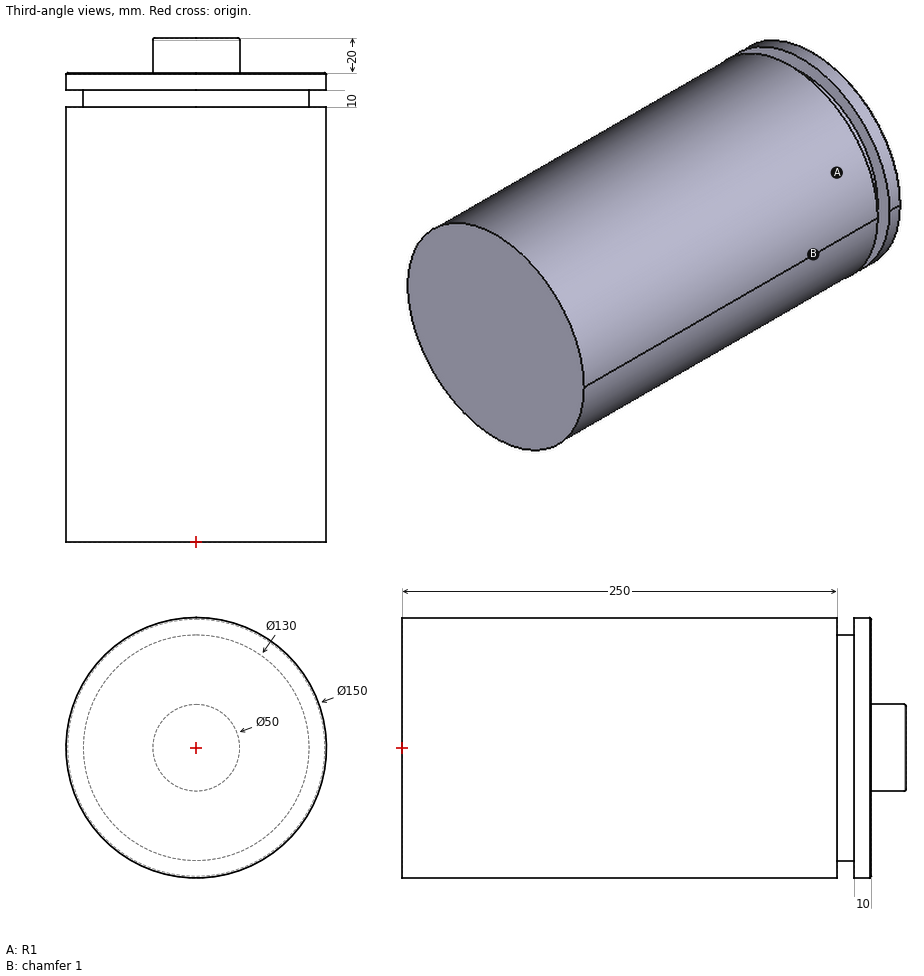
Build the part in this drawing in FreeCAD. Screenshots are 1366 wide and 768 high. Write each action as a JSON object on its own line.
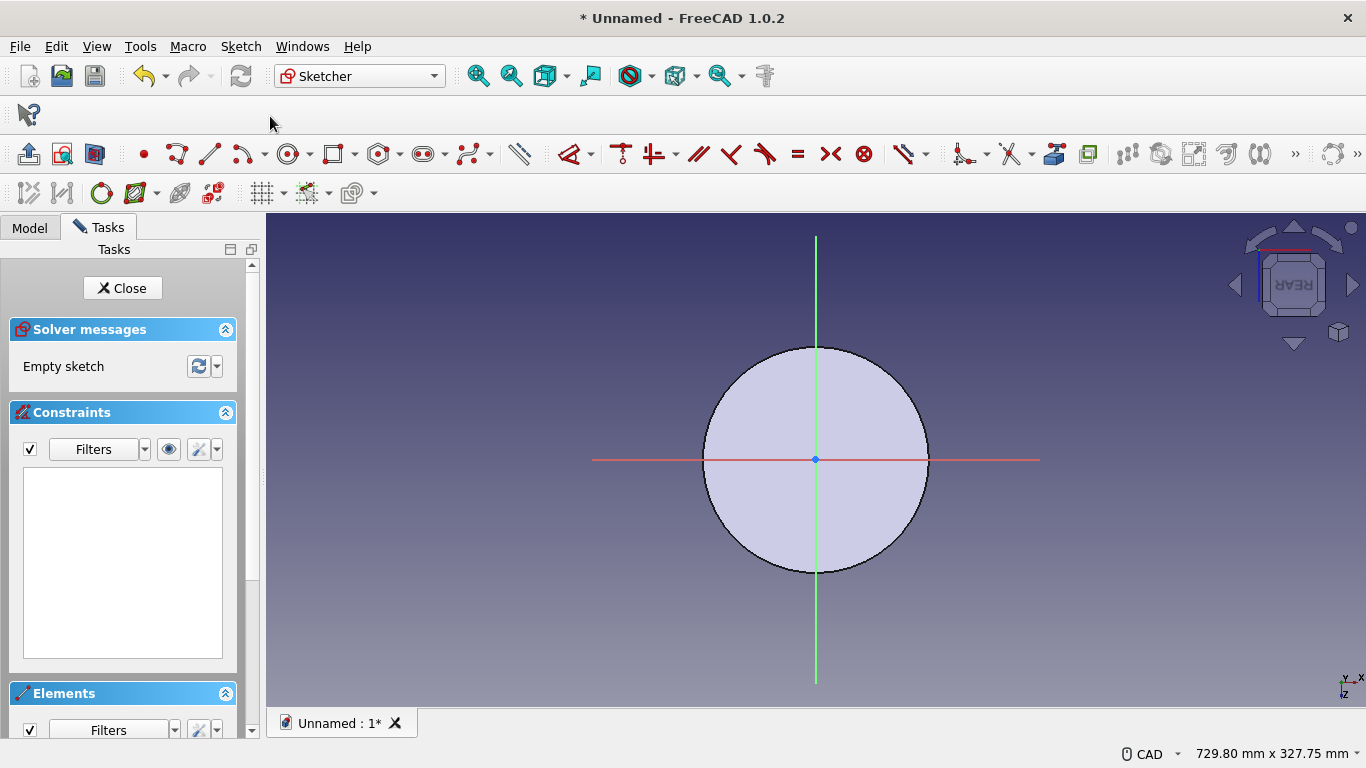
{"action": "scroll", "coordinate": [838, 460], "scroll_direction": "up", "scroll_amount": 7}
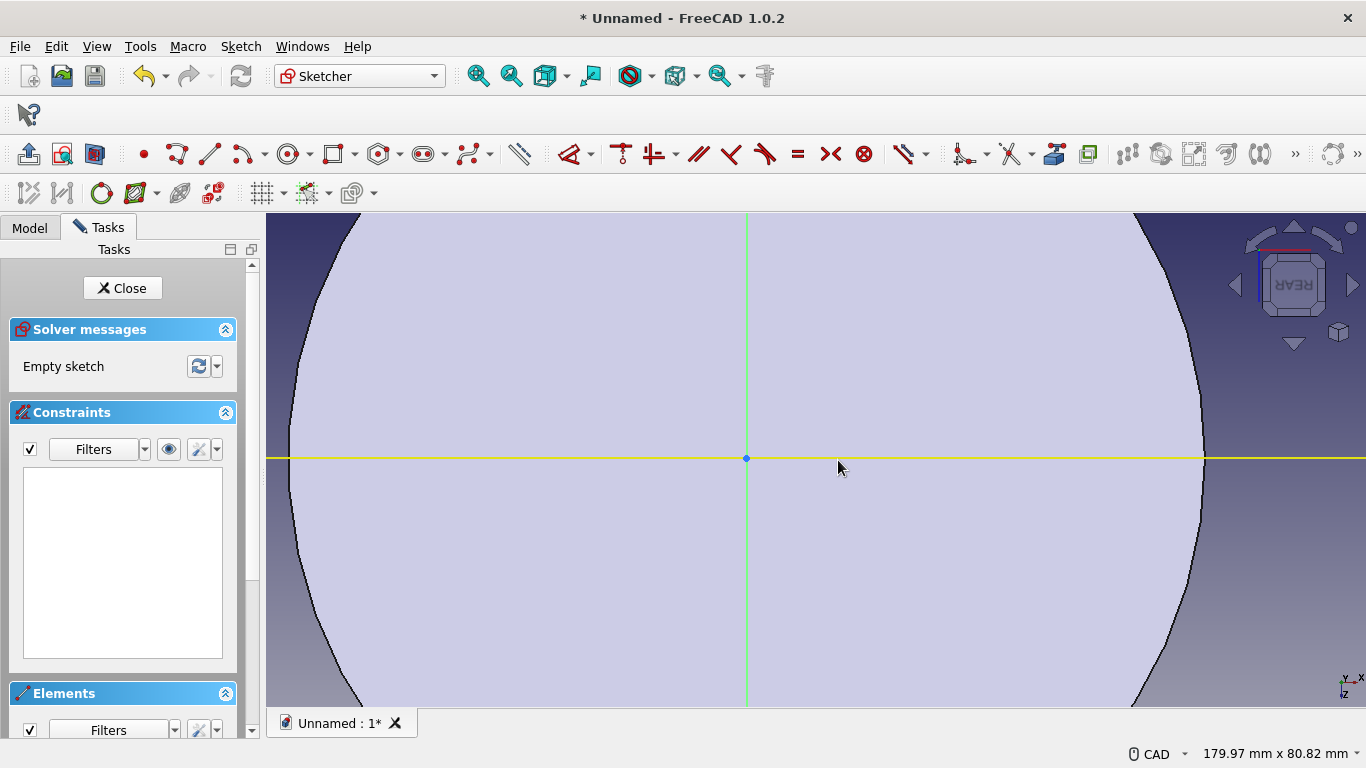
{"action": "key", "text": "g c"}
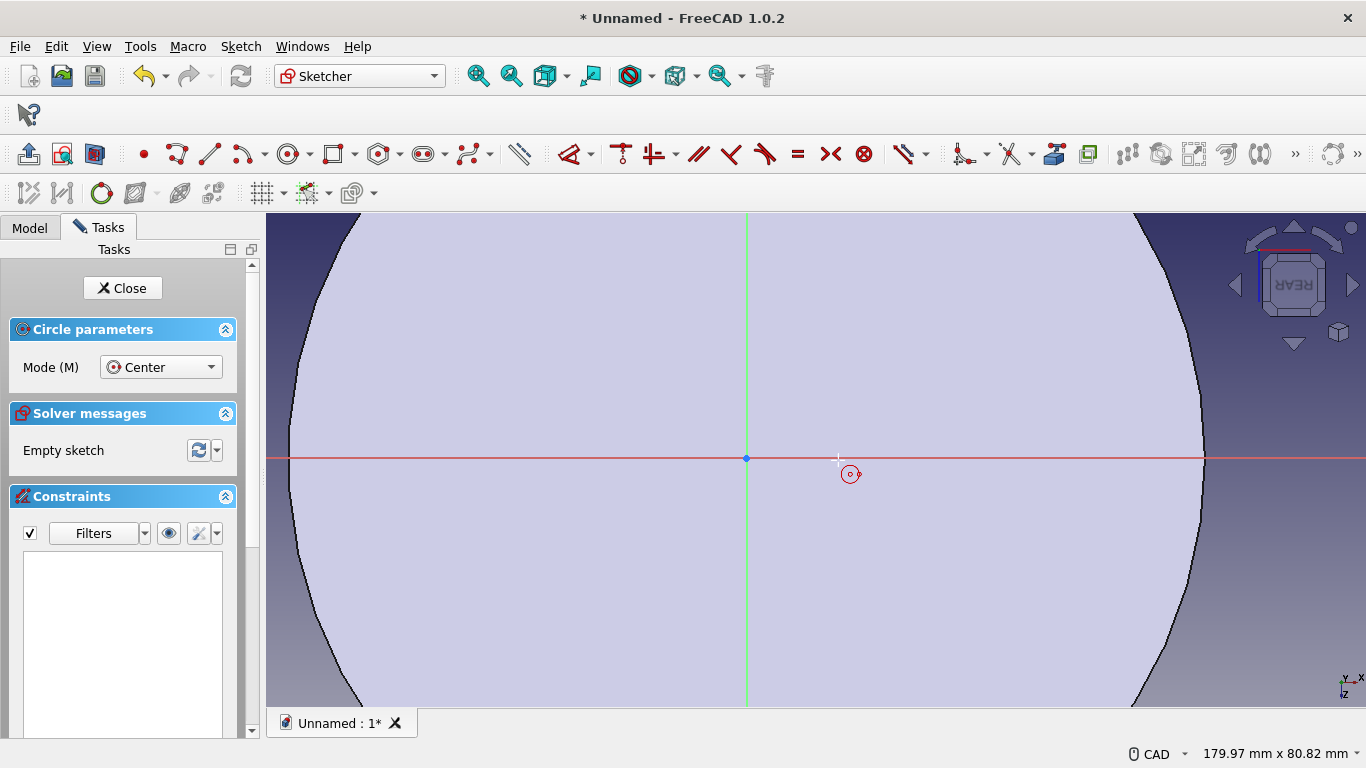
{"action": "left_click", "coordinate": [747, 458]}
{"action": "mouse_move", "coordinate": [855, 350]}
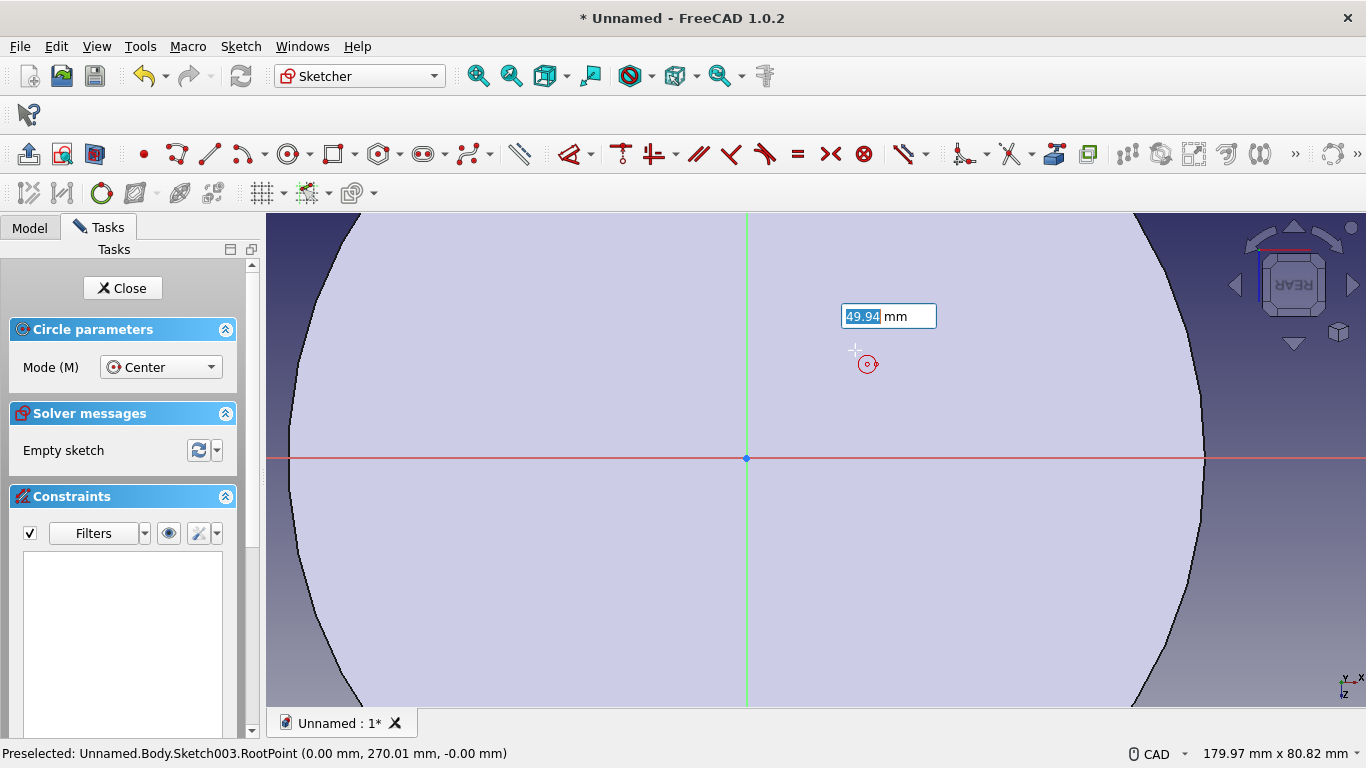
{"action": "type", "text": "50"}
{"action": "key", "text": "Return"}
{"action": "key", "text": "Escape"}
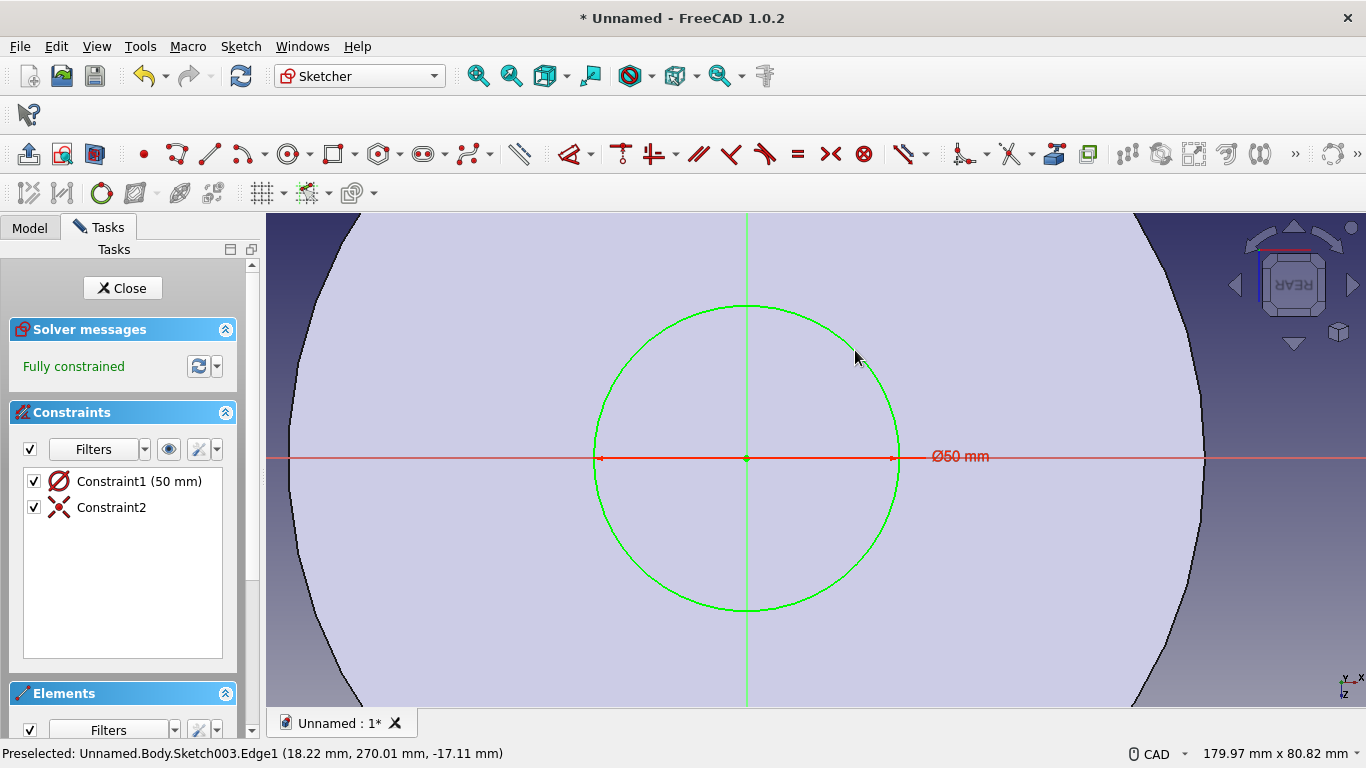
{"action": "left_click", "coordinate": [123, 288]}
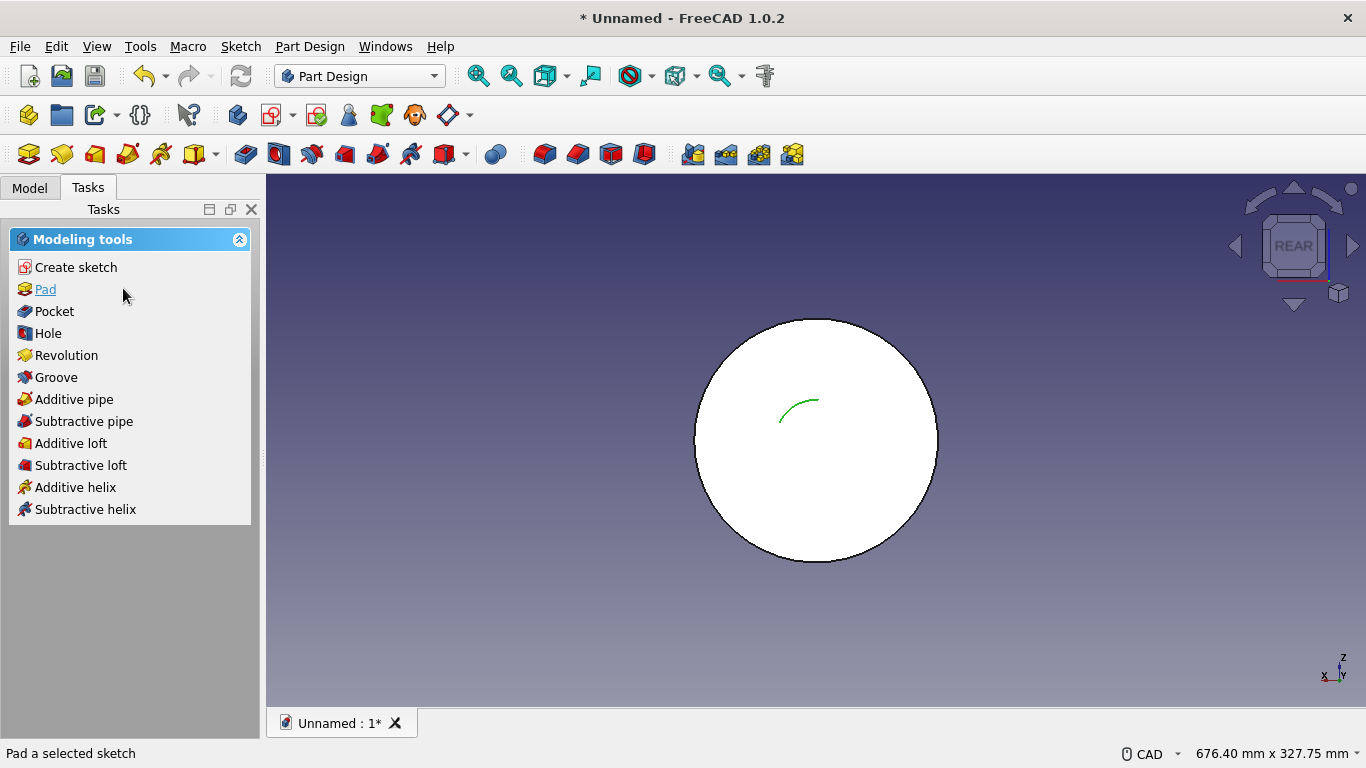
{"action": "left_click", "coordinate": [29, 154]}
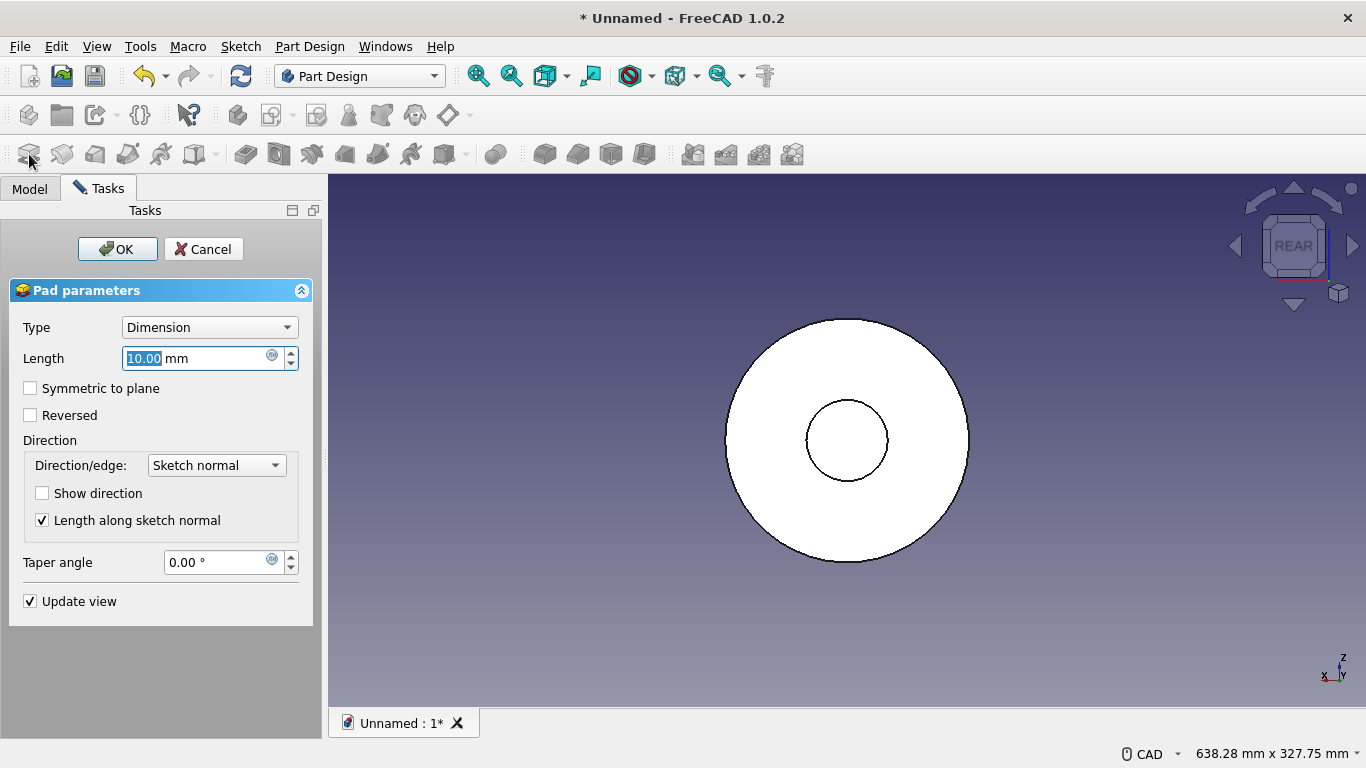
{"action": "type", "text": "20"}
{"action": "key", "text": "Tab"}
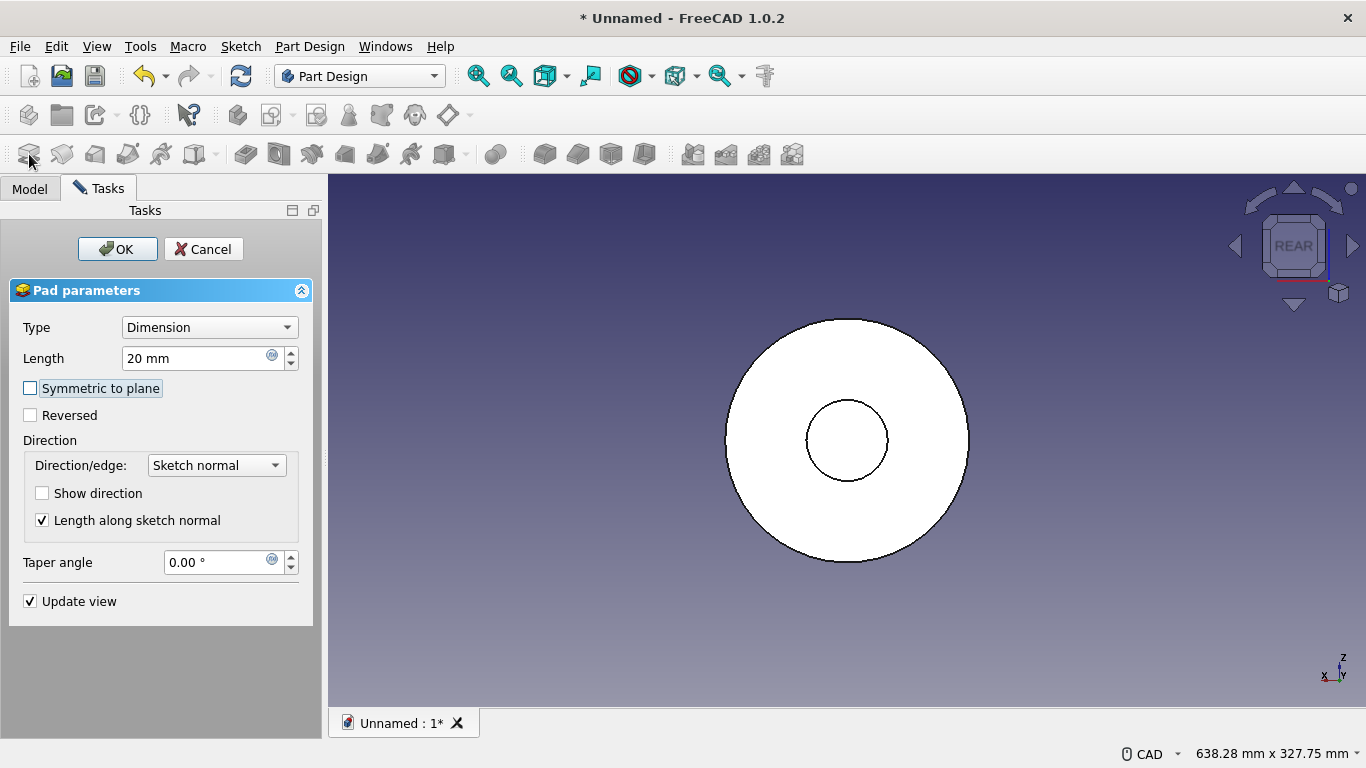
{"action": "left_click", "coordinate": [118, 249]}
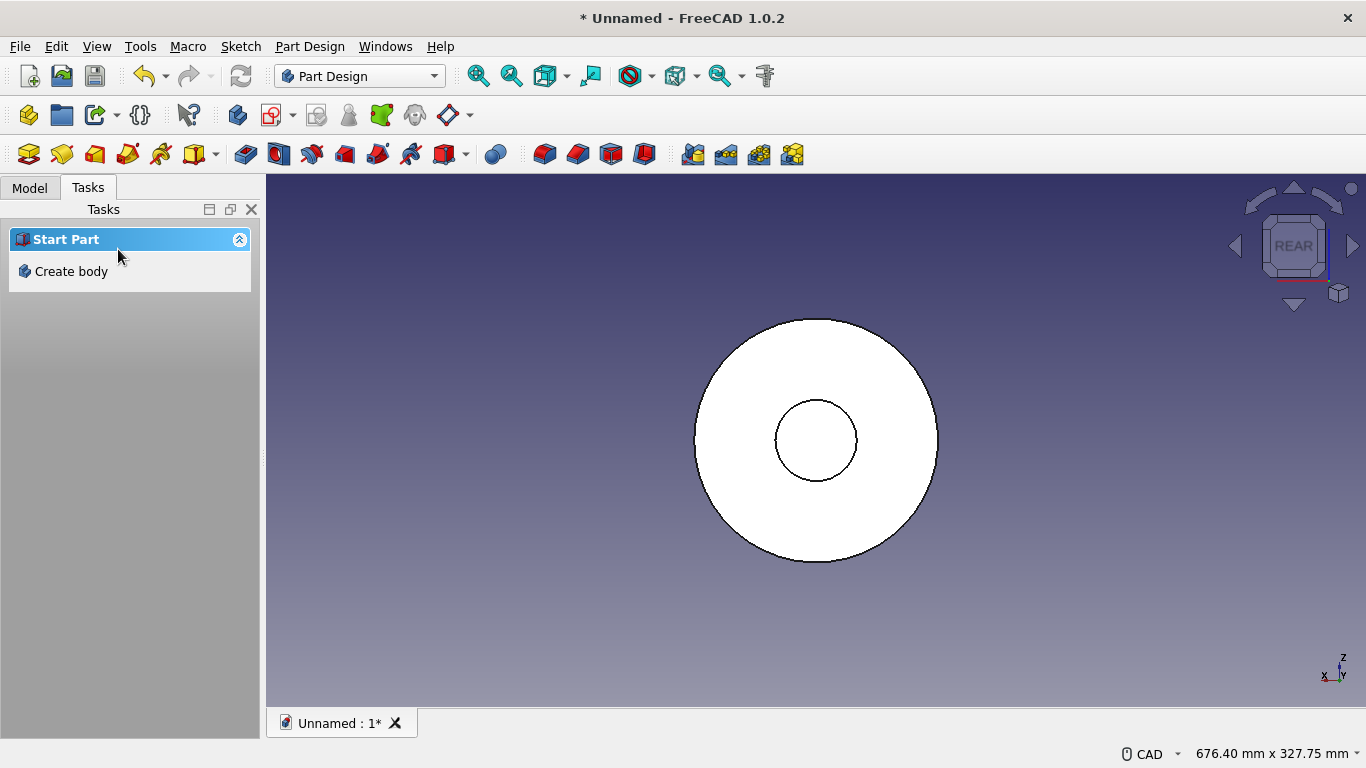
{"action": "left_click", "coordinate": [857, 440]}